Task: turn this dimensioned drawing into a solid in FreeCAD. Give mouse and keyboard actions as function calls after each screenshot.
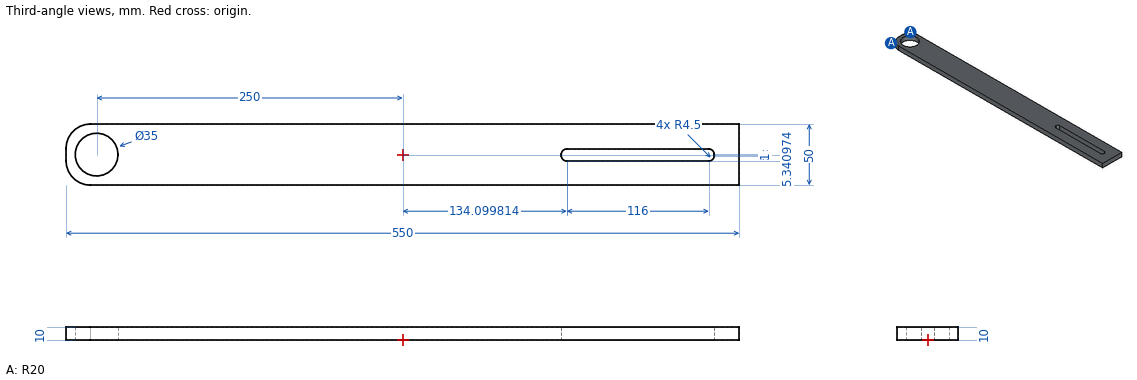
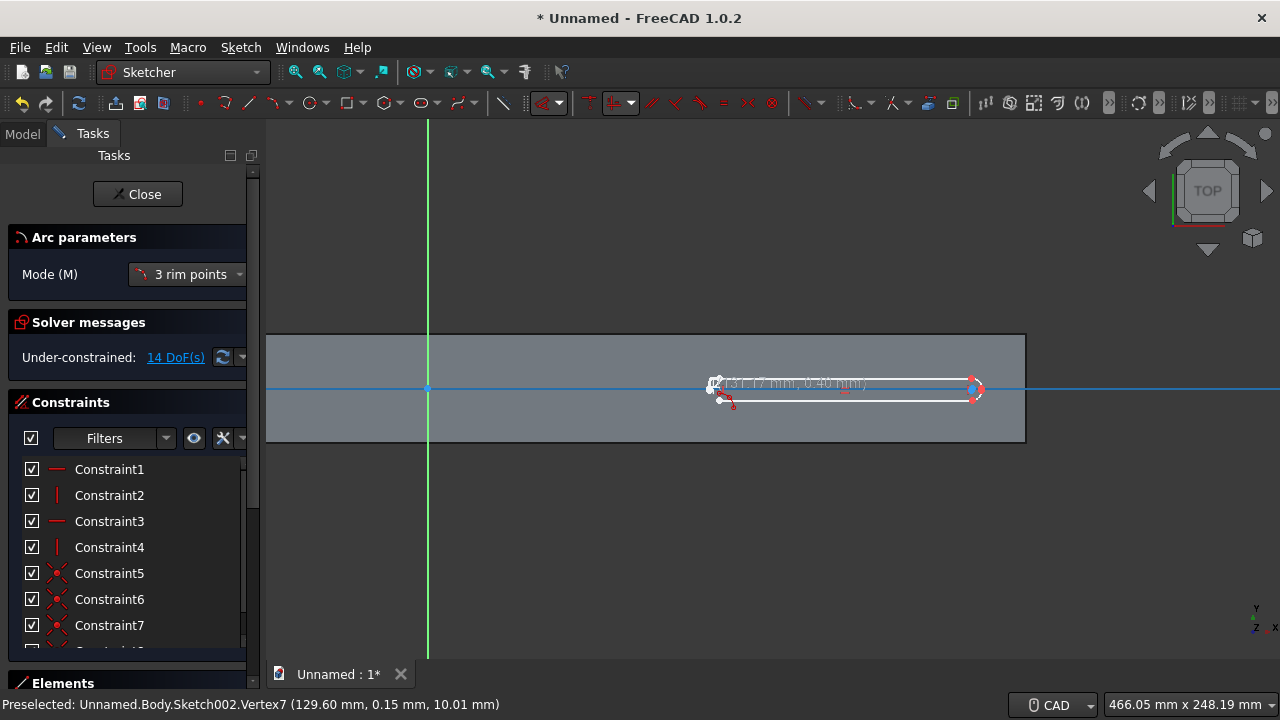
scroll(713, 381, up, 9)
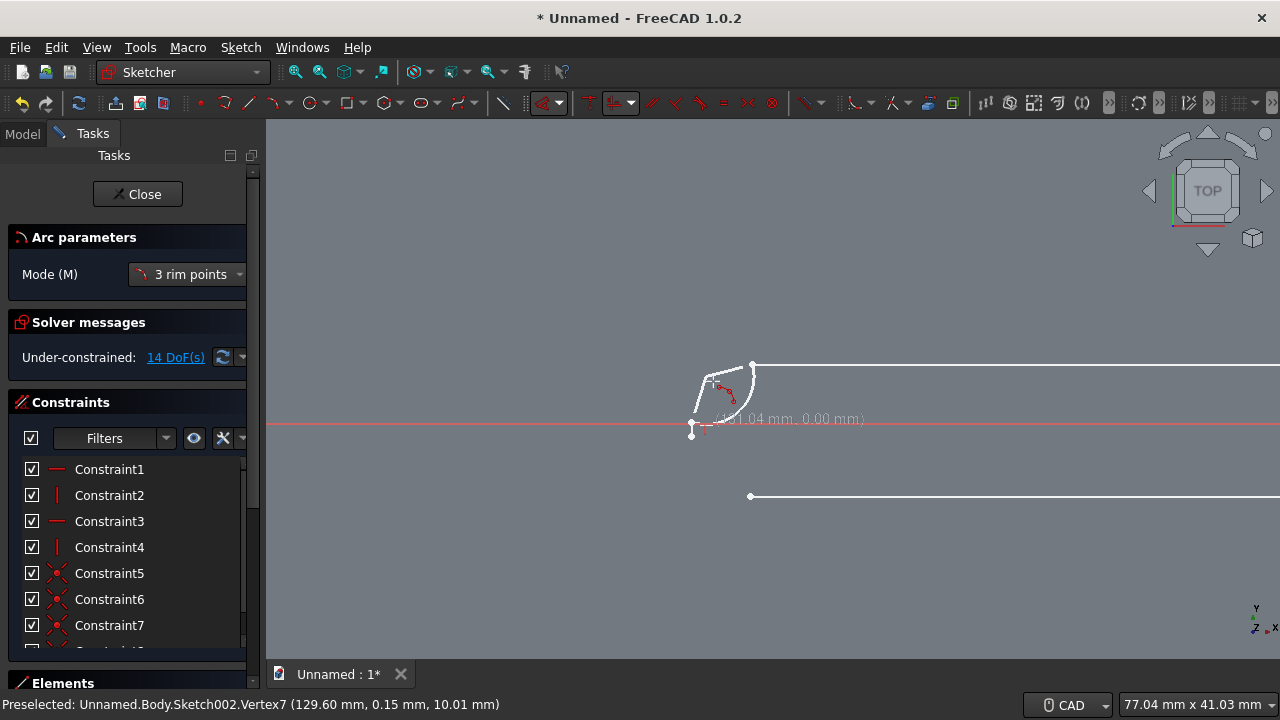
click(709, 380)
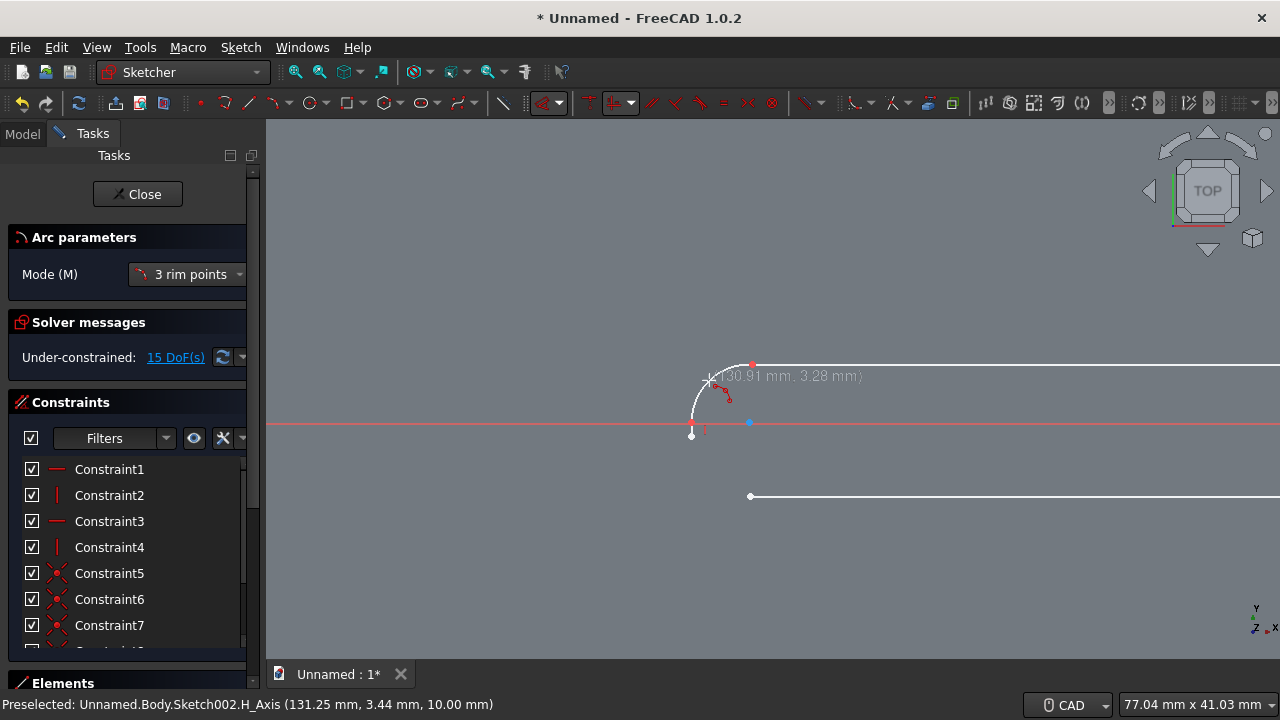
scroll(692, 435, up, 5)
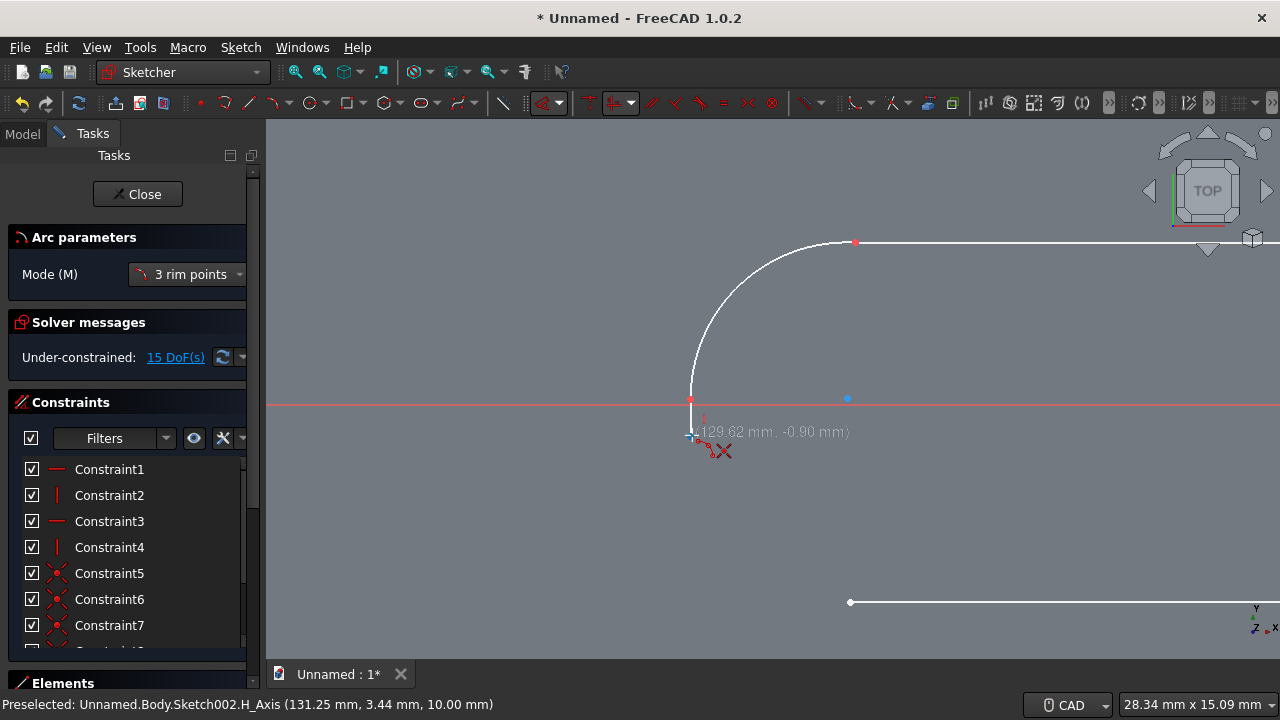
click(691, 437)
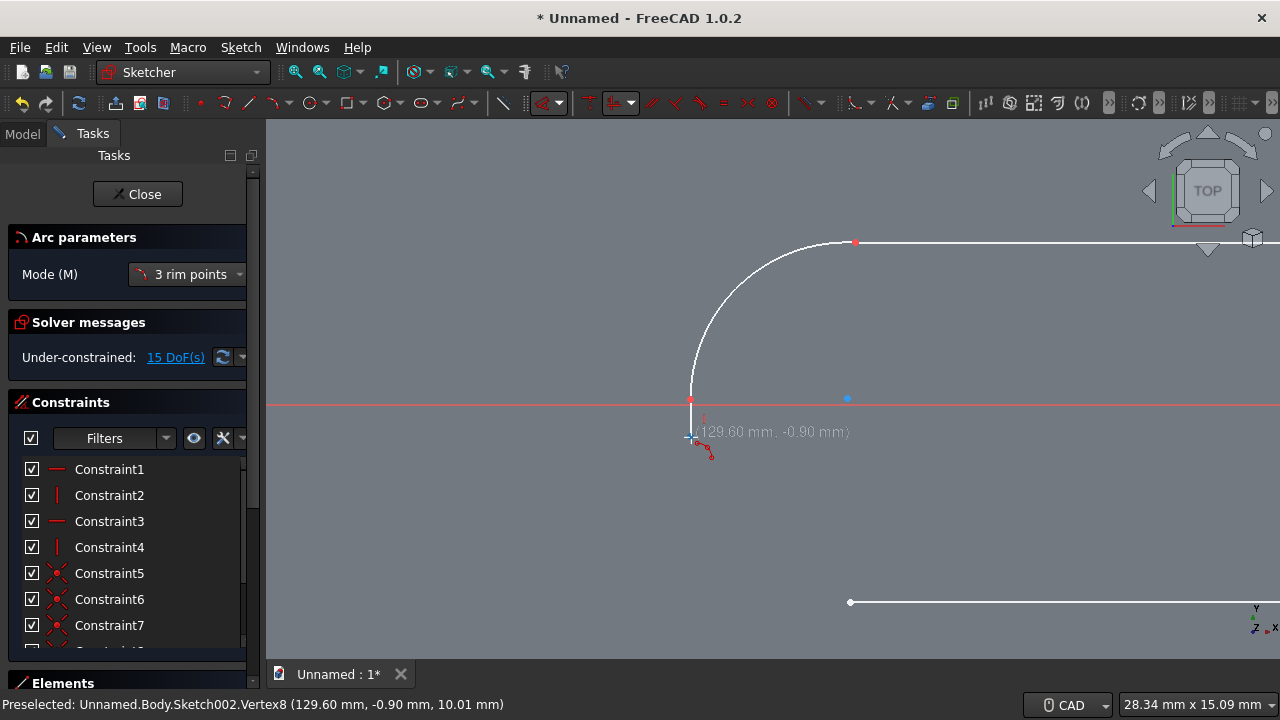
scroll(711, 387, down, 14)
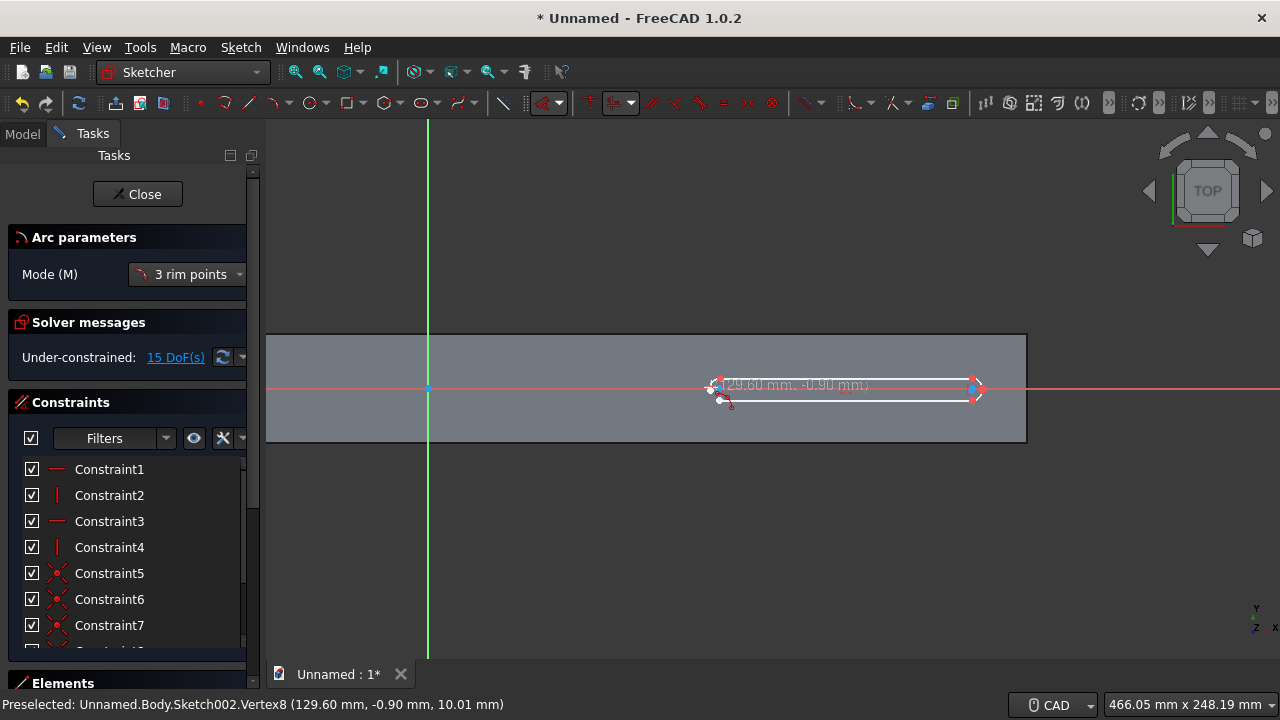
scroll(720, 400, up, 2)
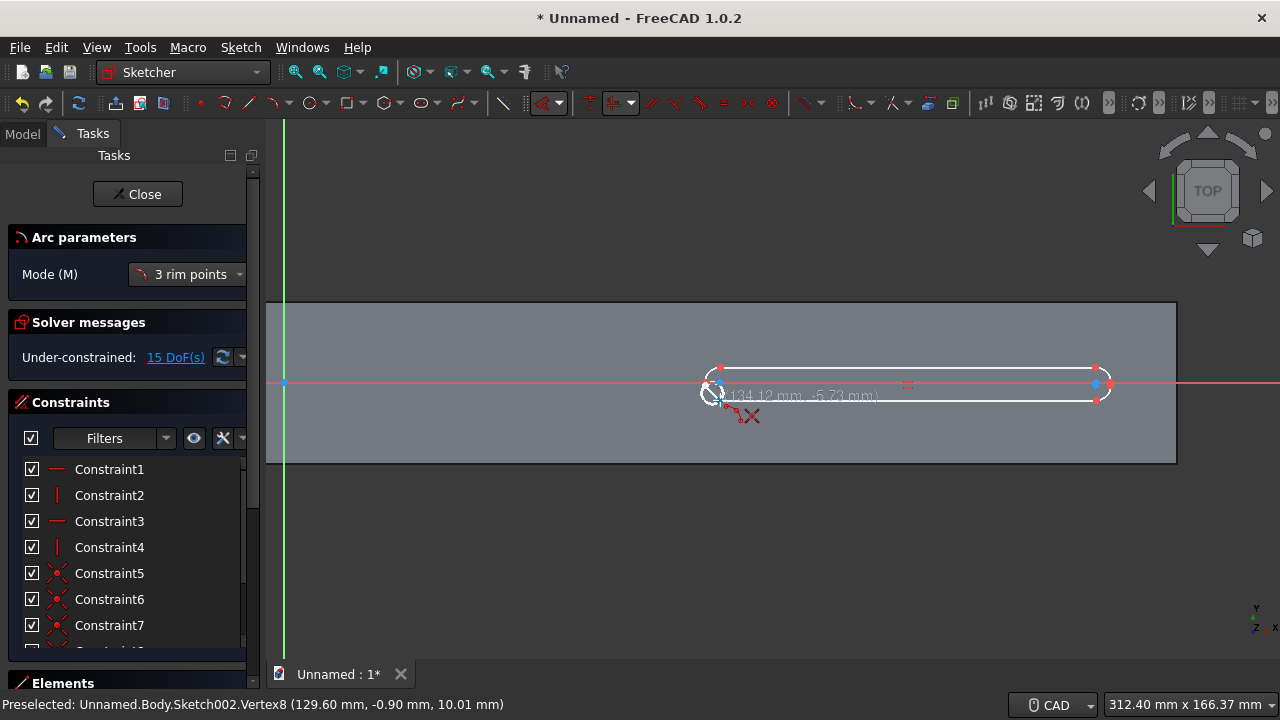
click(720, 401)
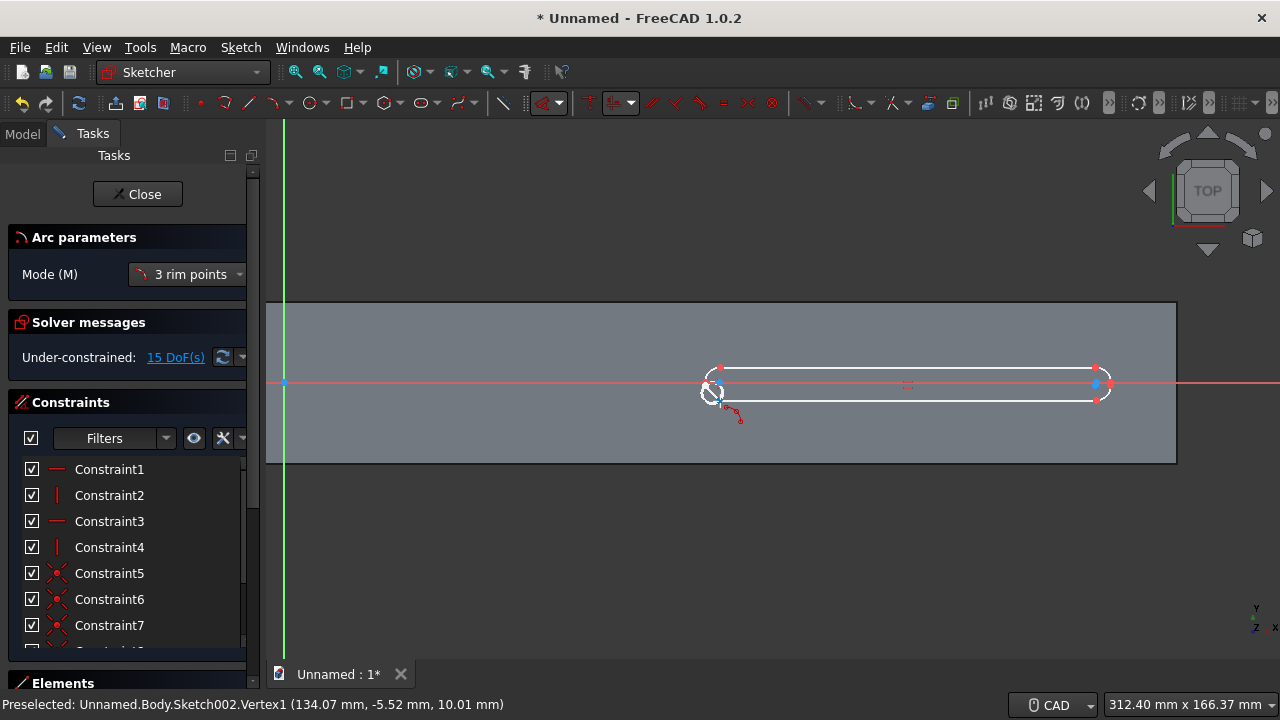
scroll(709, 396, up, 7)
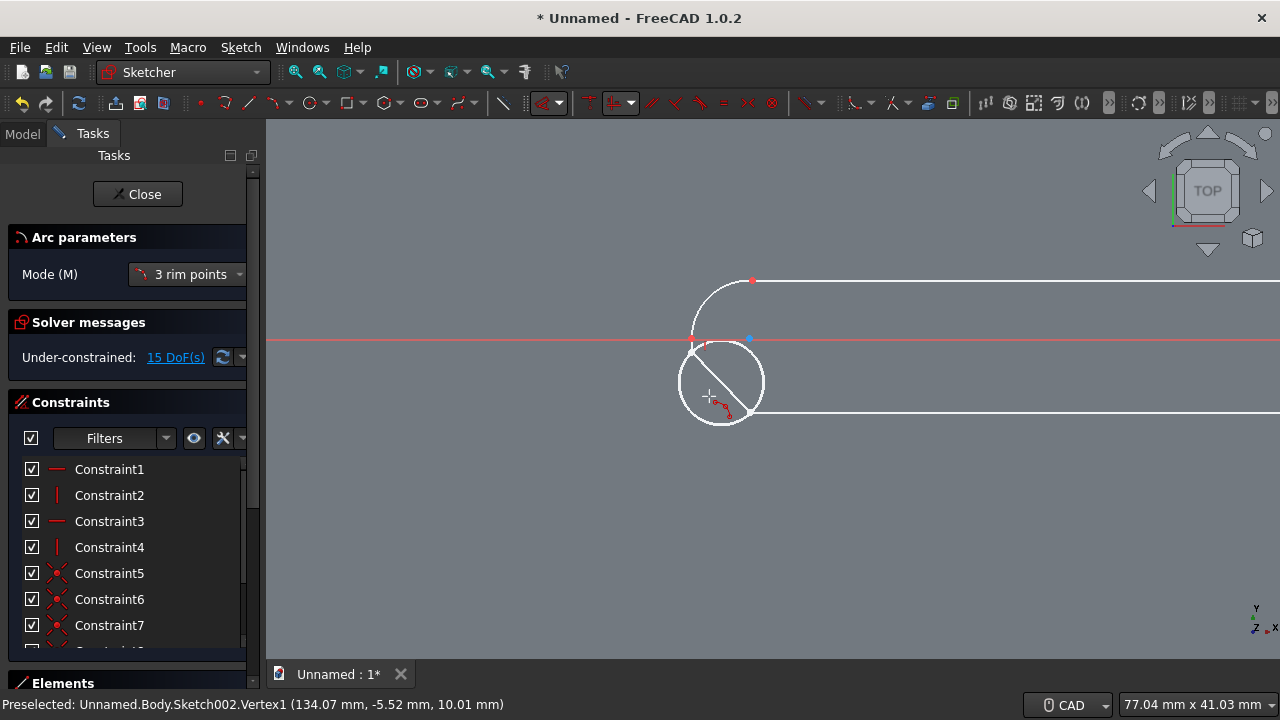
click(709, 393)
key(Escape)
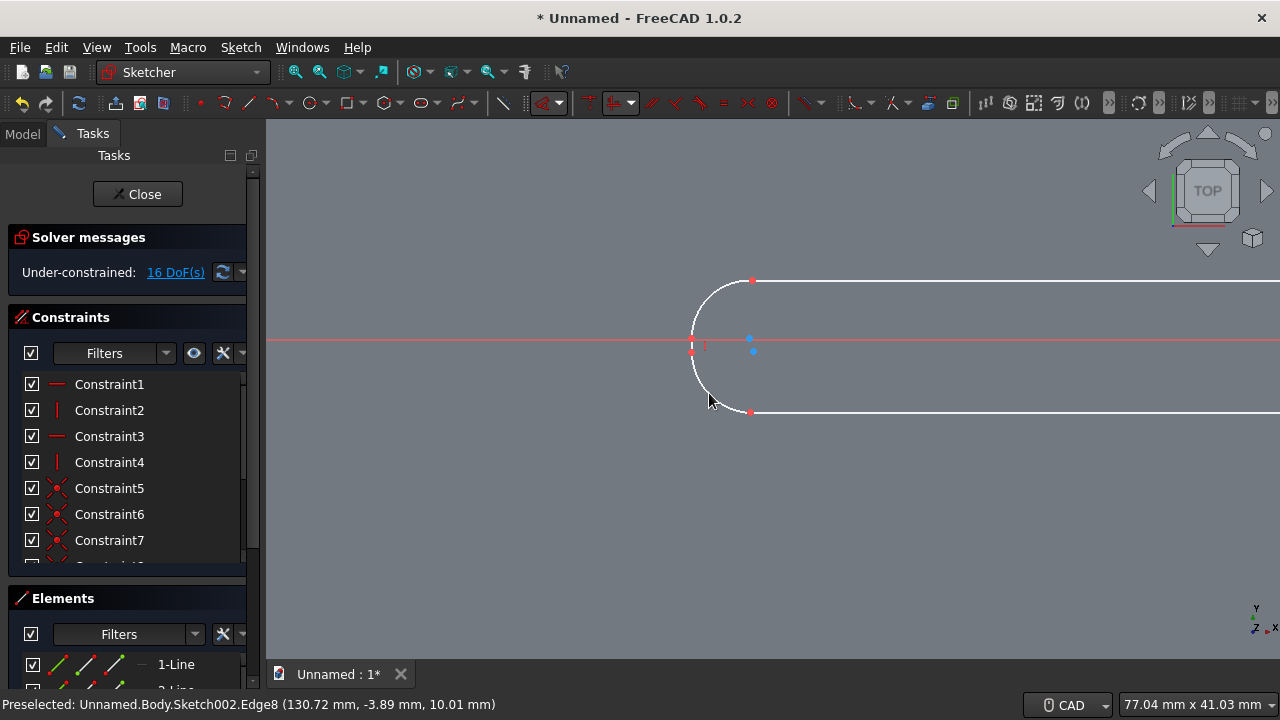
scroll(713, 398, down, 9)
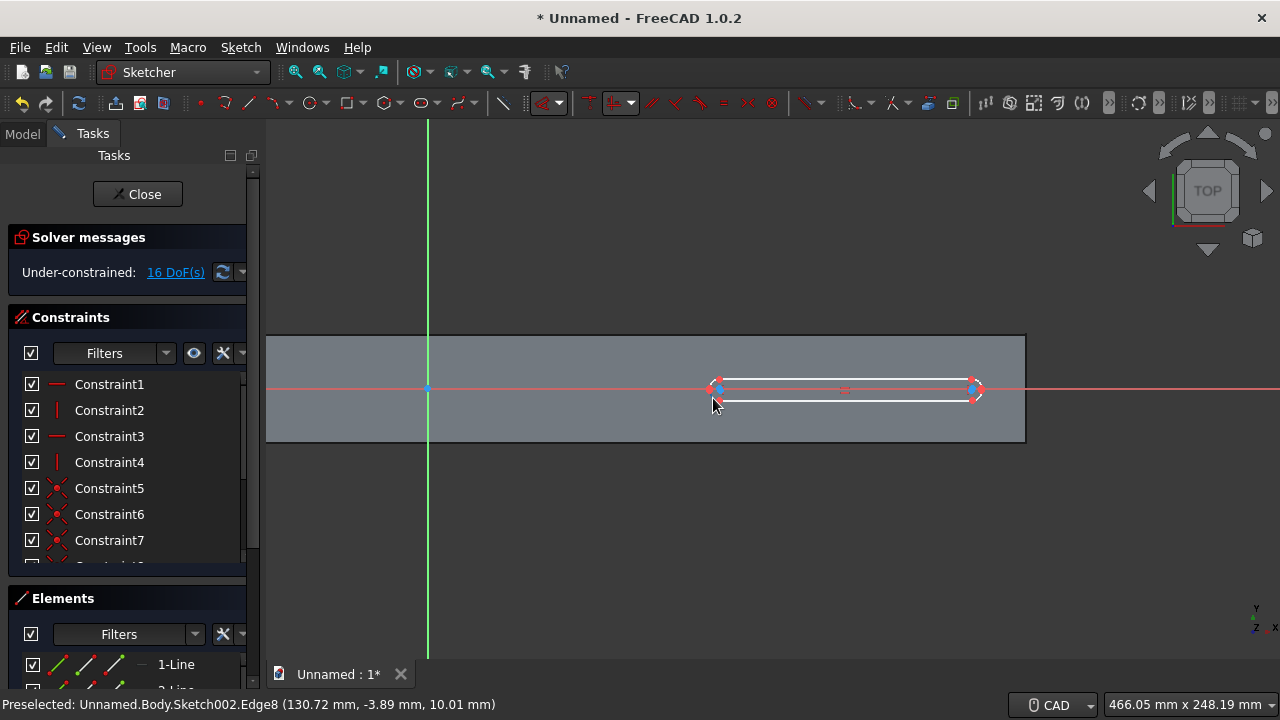
click(770, 401)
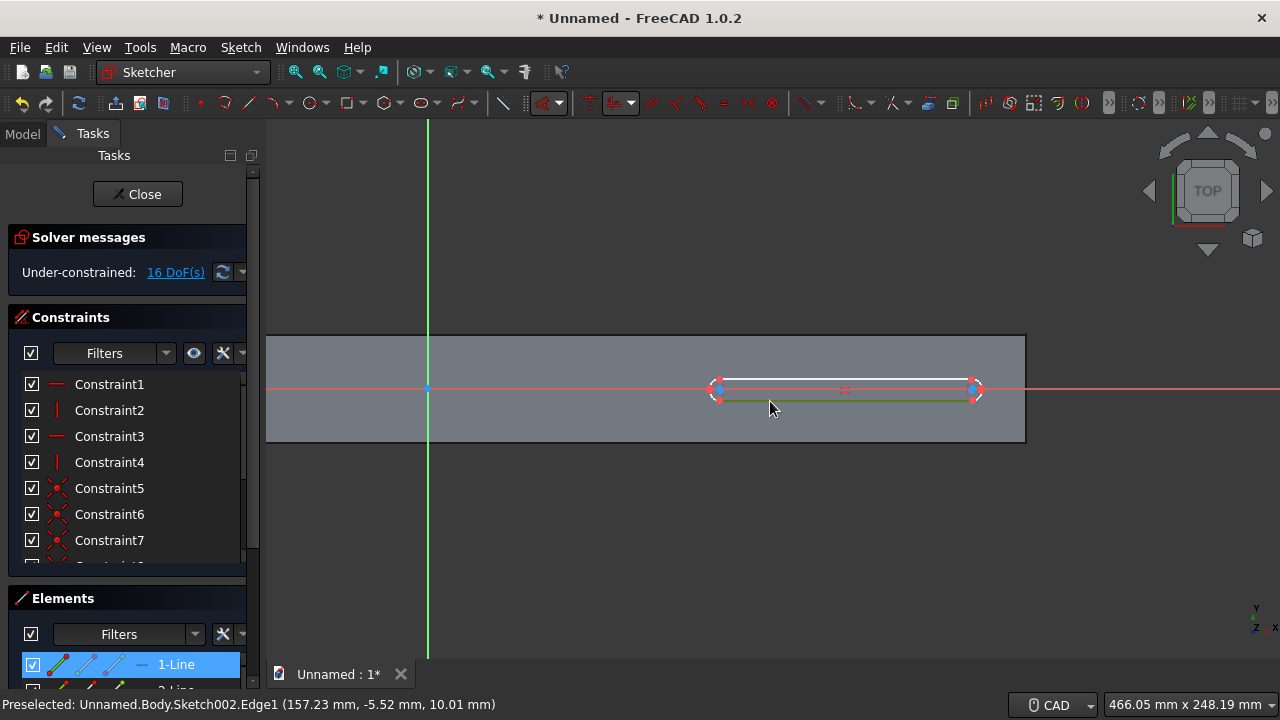
scroll(979, 398, up, 4)